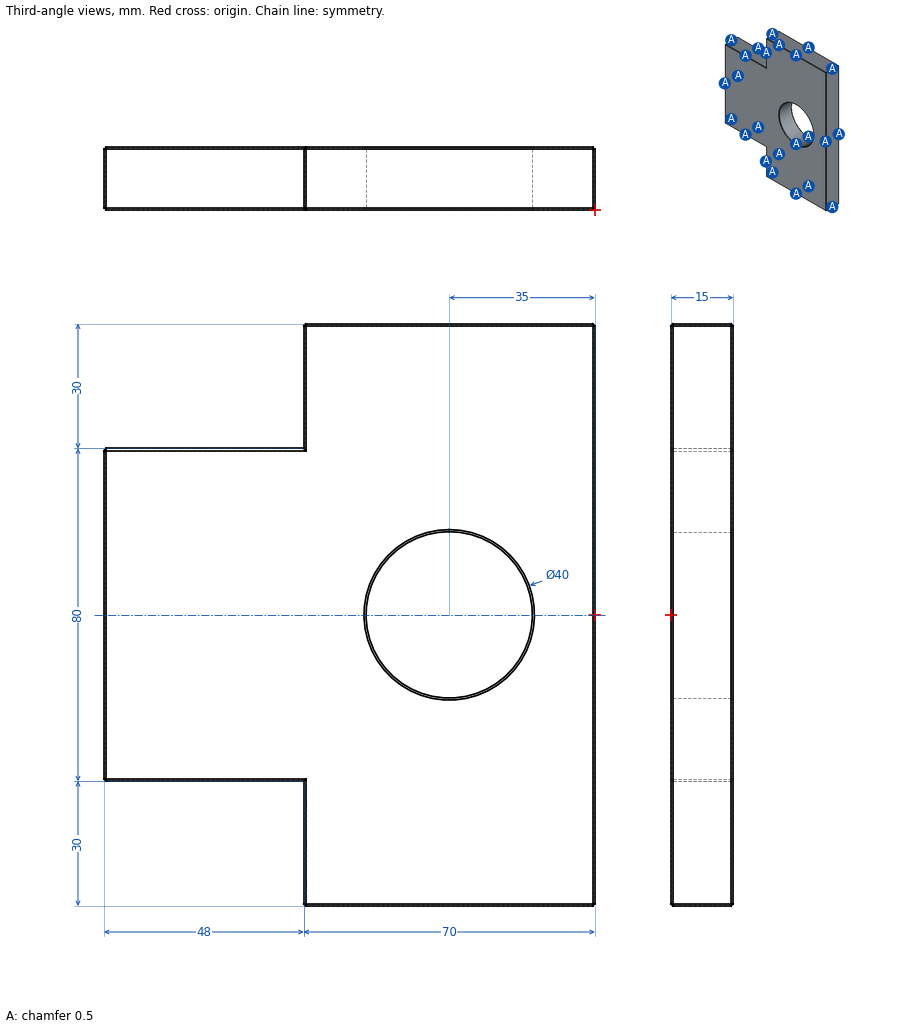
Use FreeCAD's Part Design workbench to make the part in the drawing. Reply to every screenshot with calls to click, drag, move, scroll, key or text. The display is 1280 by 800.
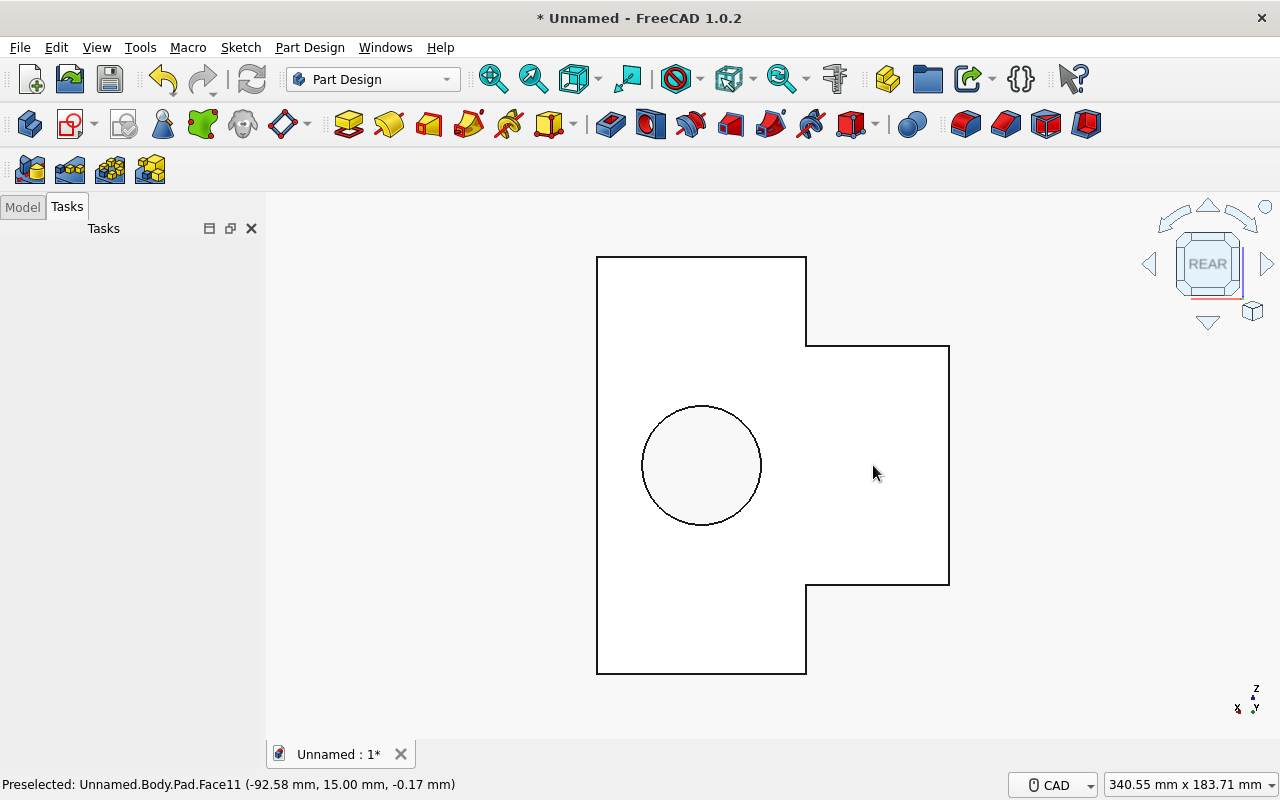
click(1006, 124)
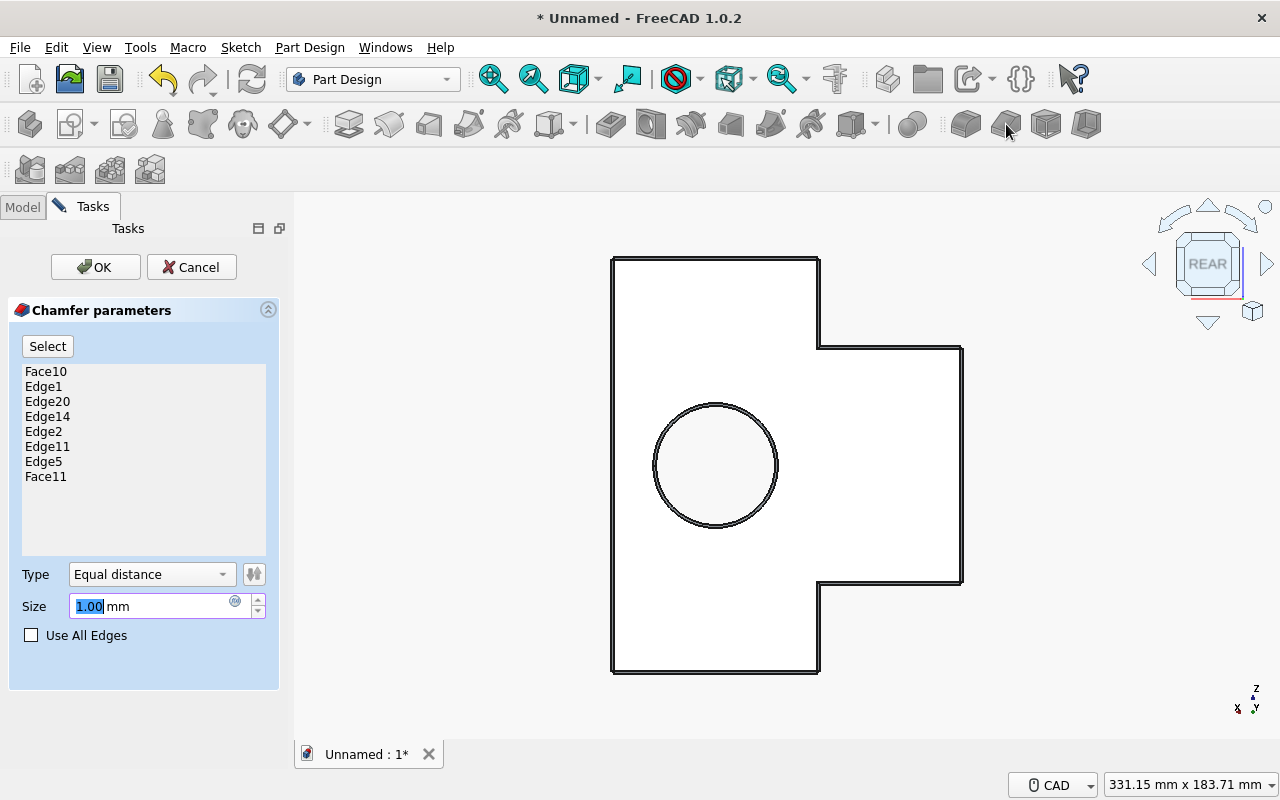
text(0.5)
key(Tab)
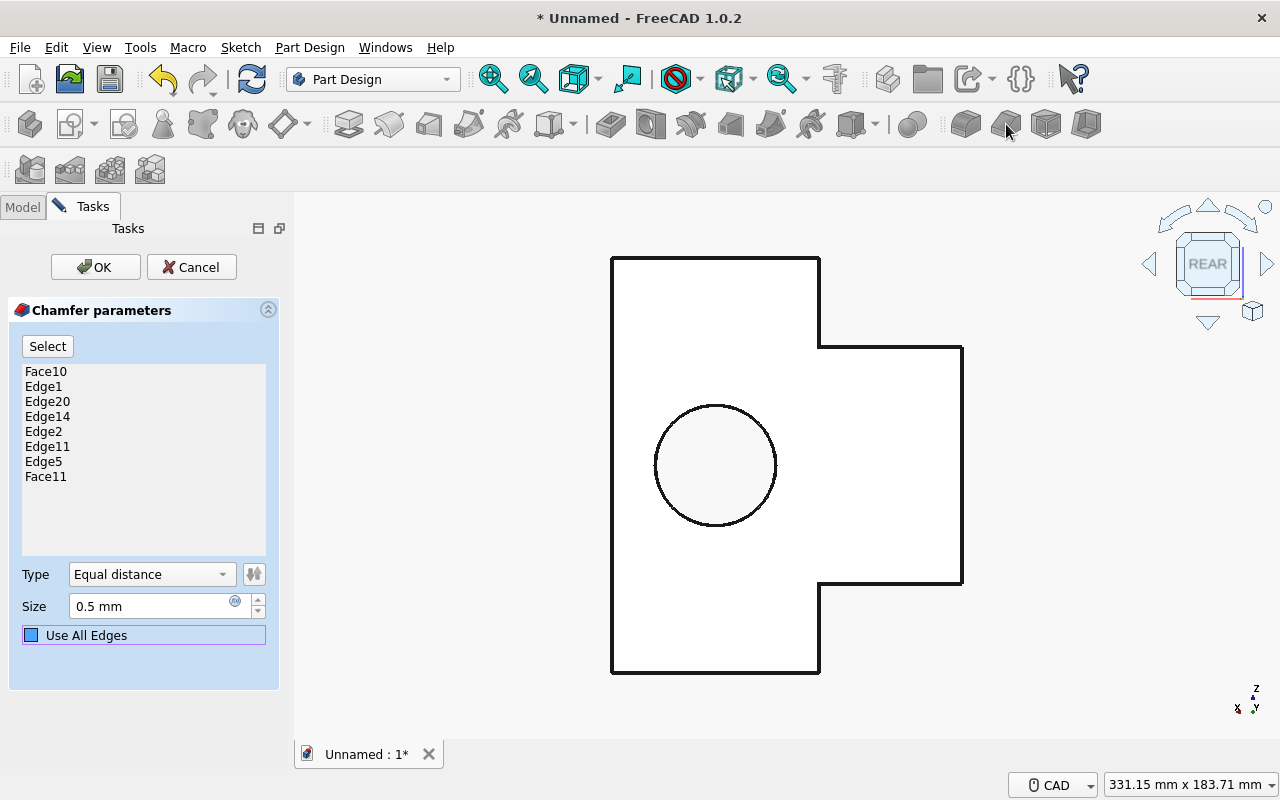
click(96, 267)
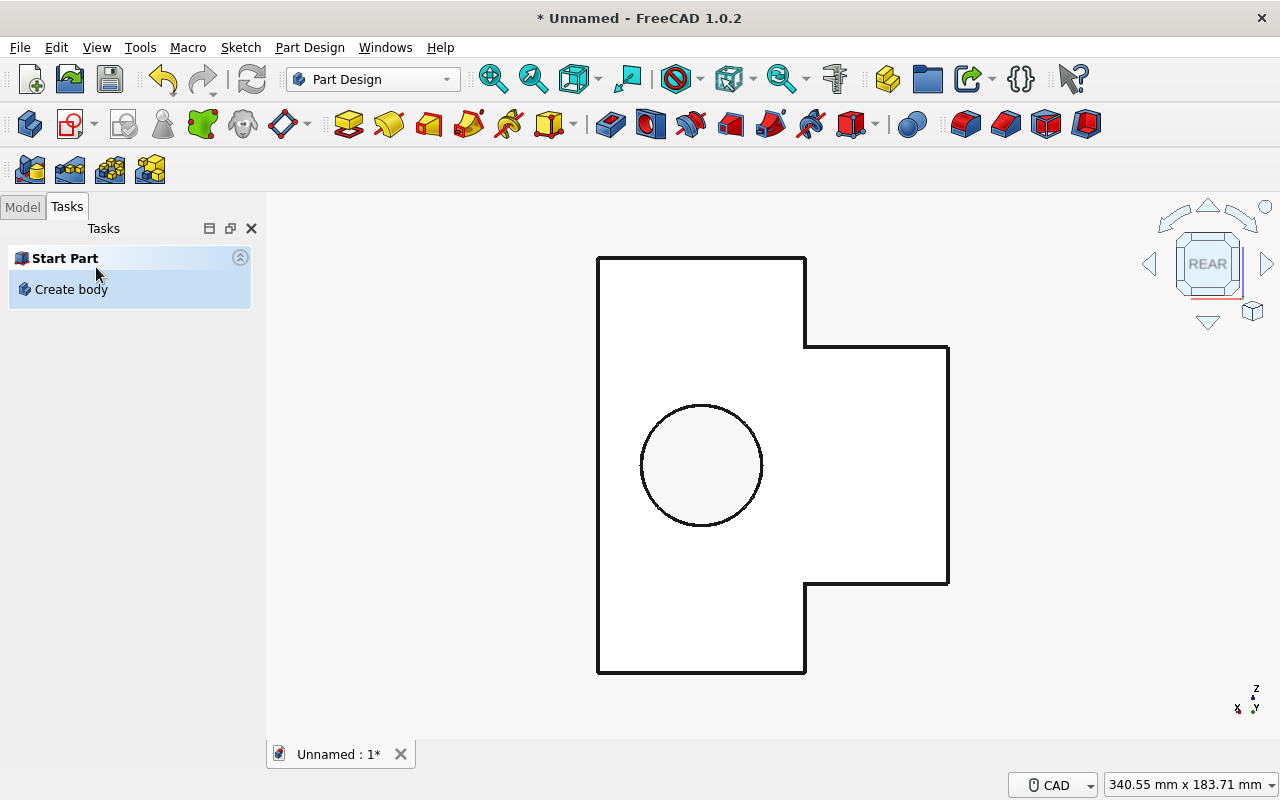
key(0)